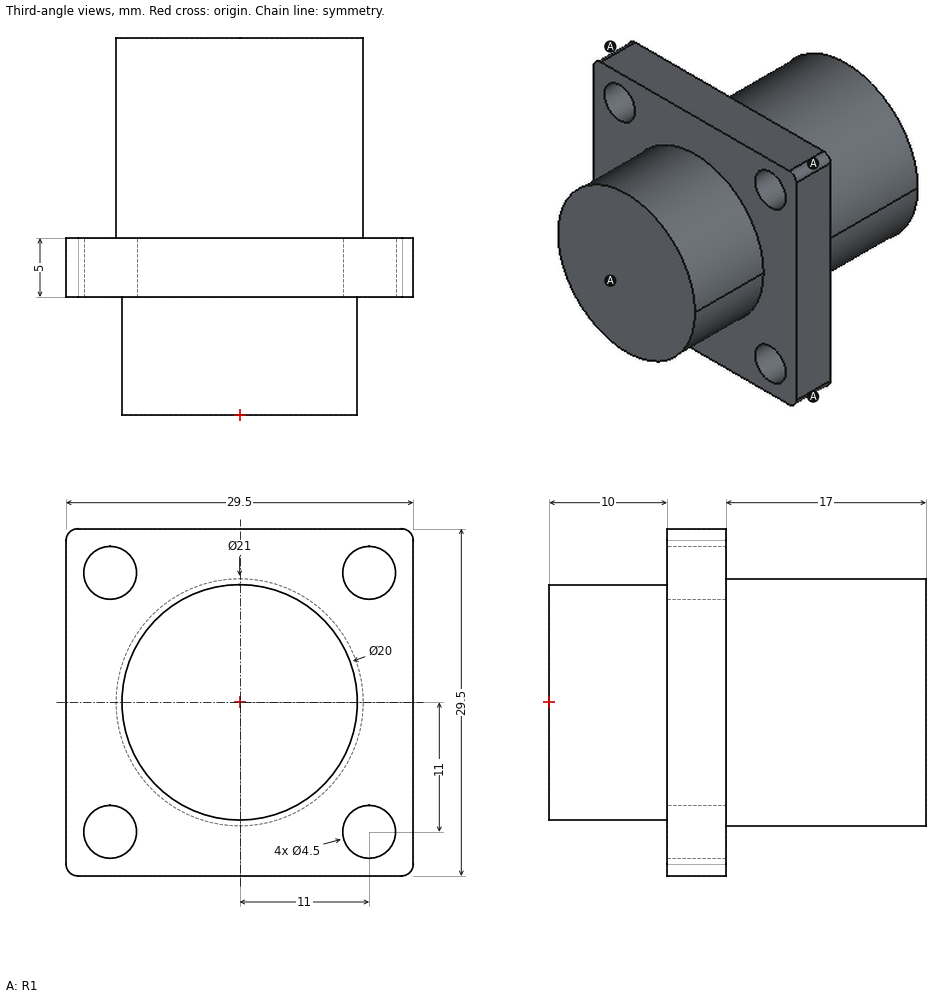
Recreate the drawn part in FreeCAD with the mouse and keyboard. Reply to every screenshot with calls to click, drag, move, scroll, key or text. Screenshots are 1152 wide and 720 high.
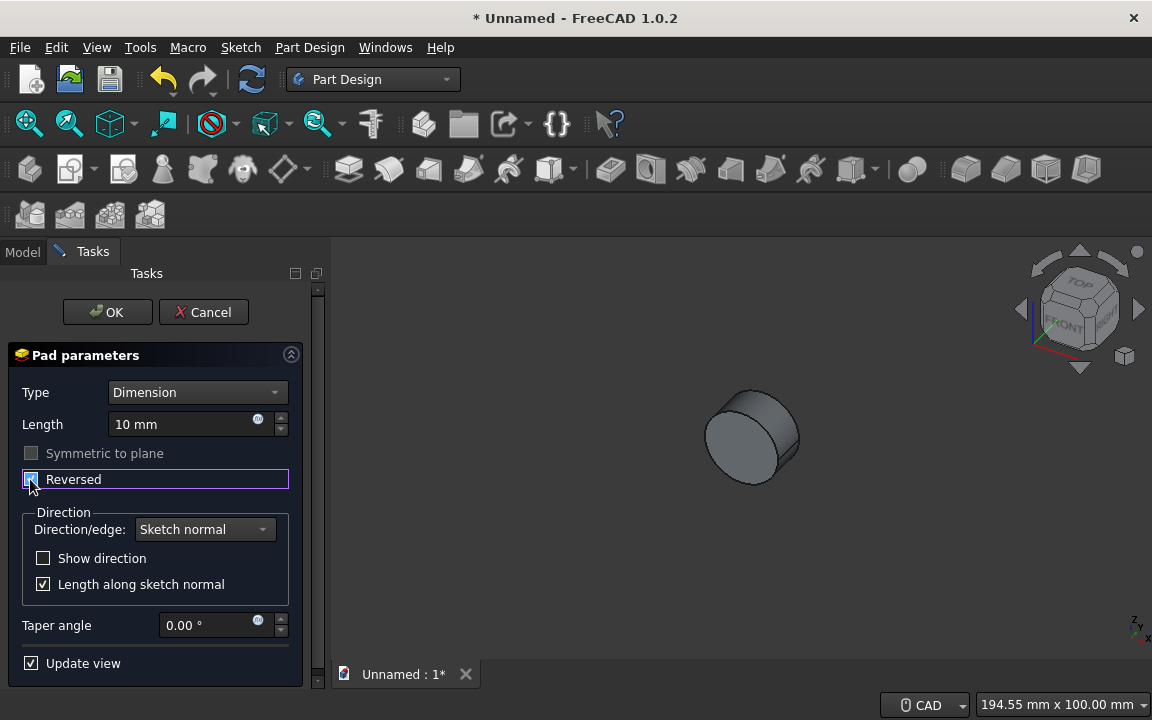
click(108, 312)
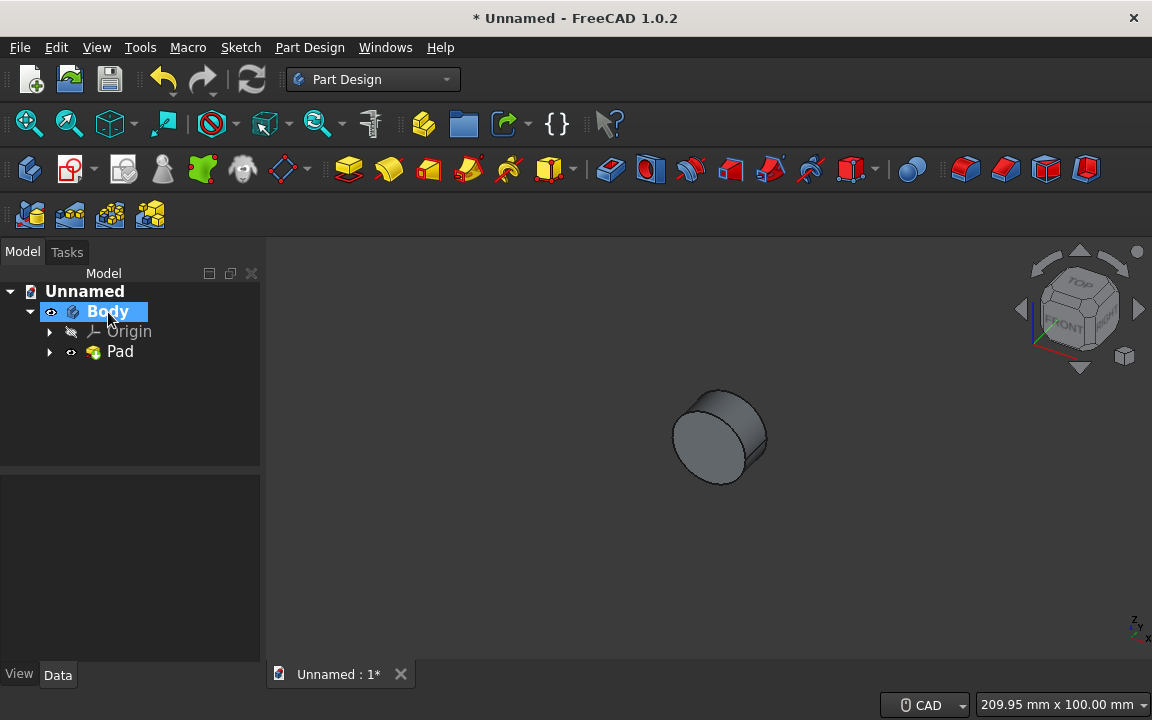
key(v)
key(f)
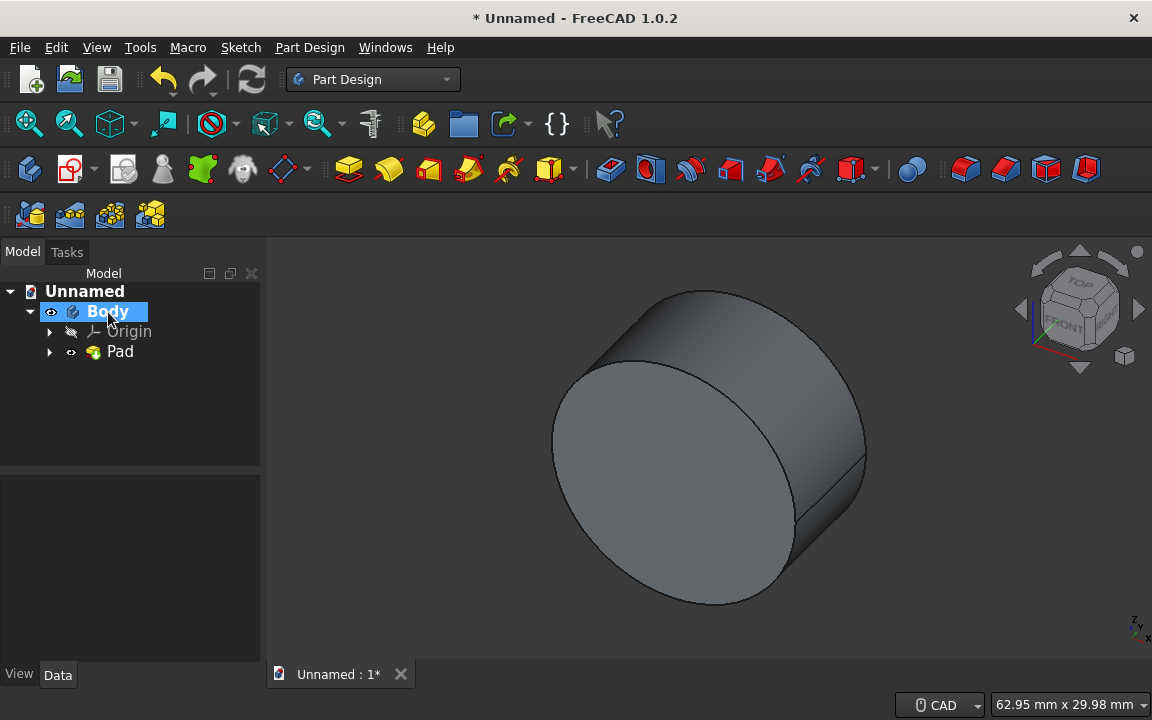
key(4)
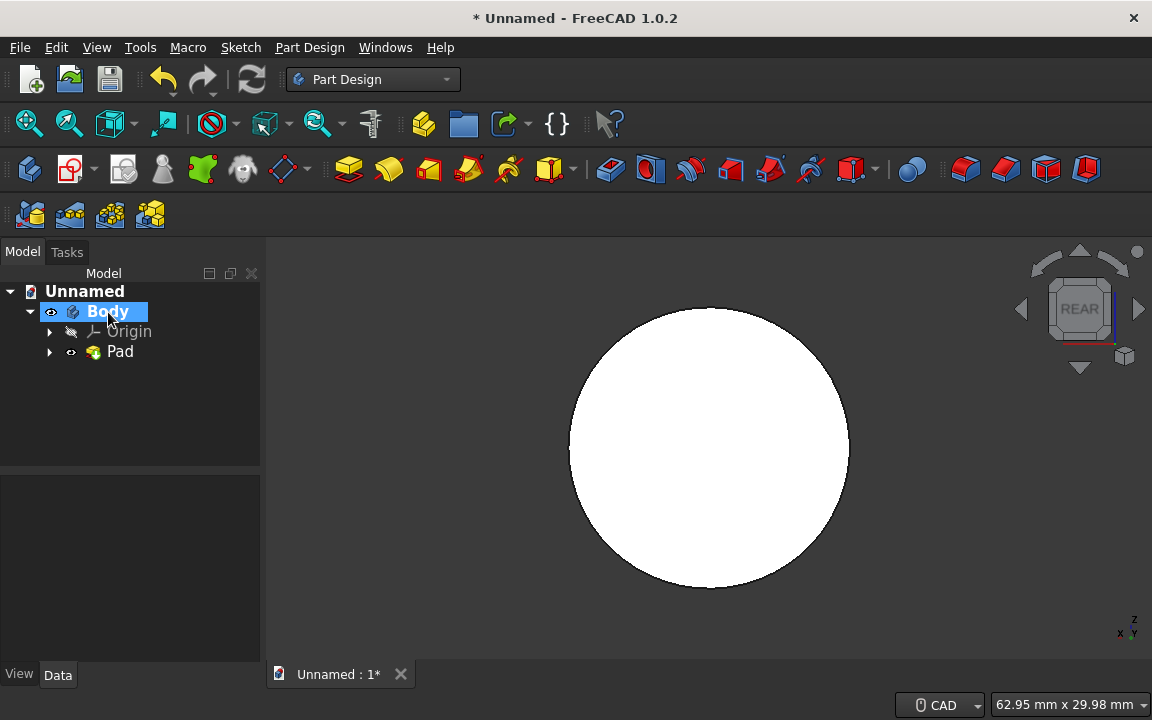
click(709, 447)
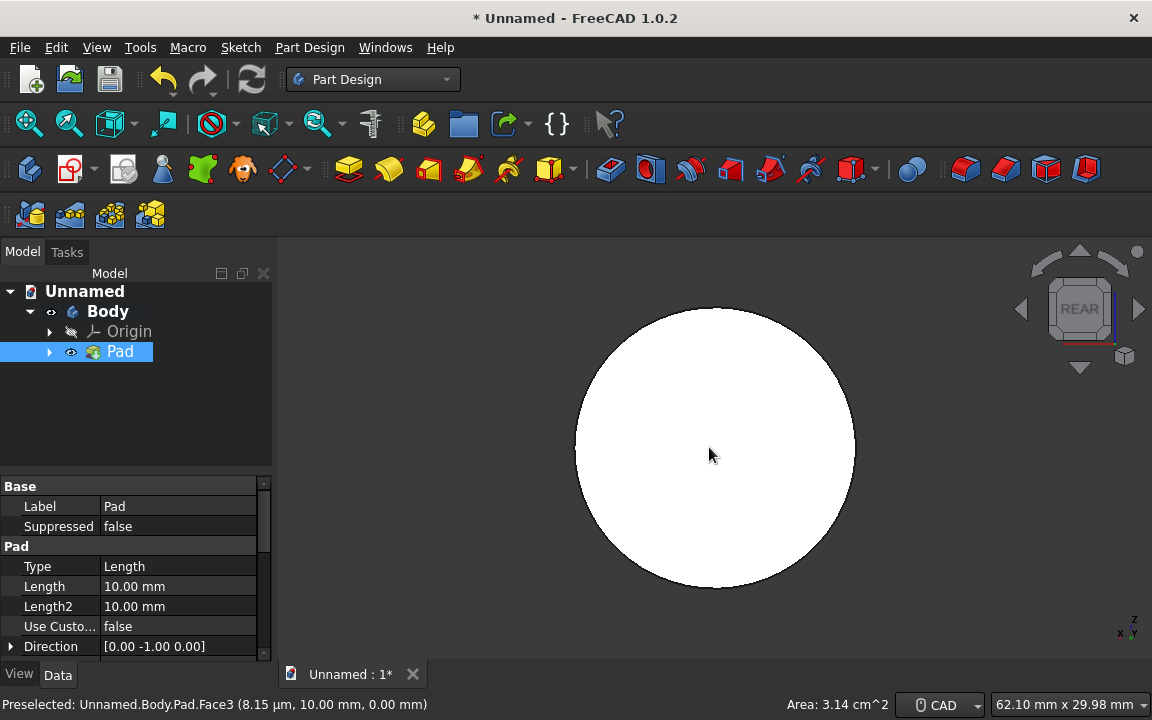
click(70, 170)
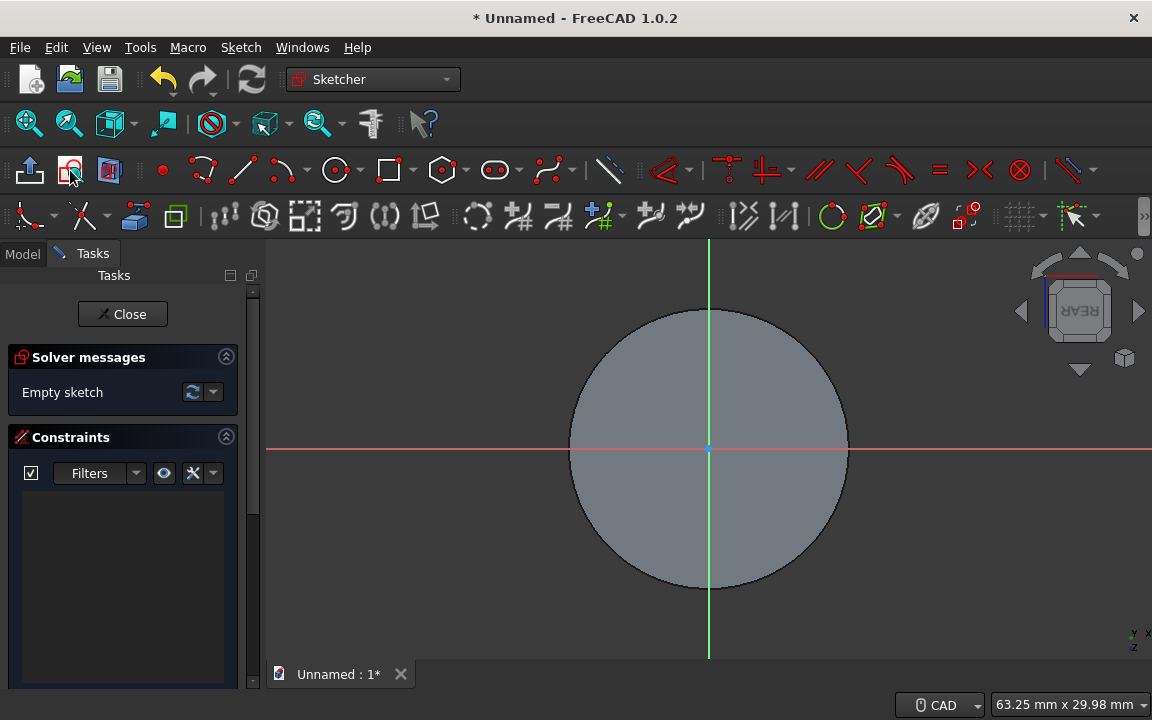
scroll(501, 449, down, 2)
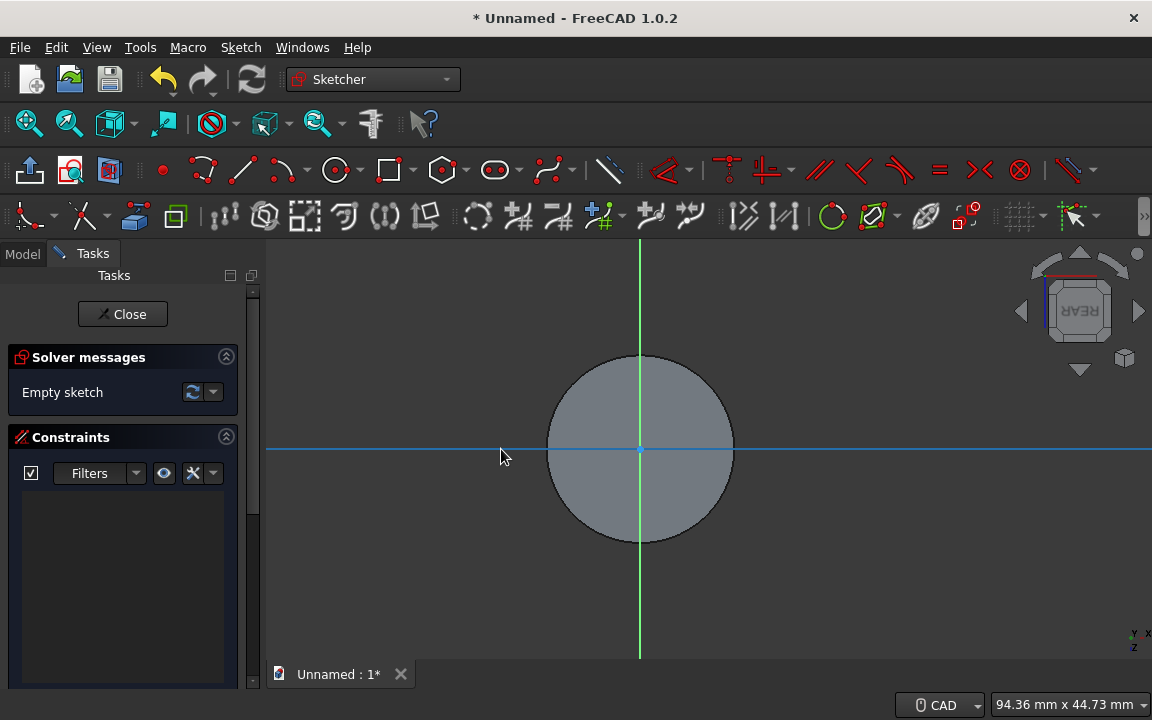
key(g)
key(v)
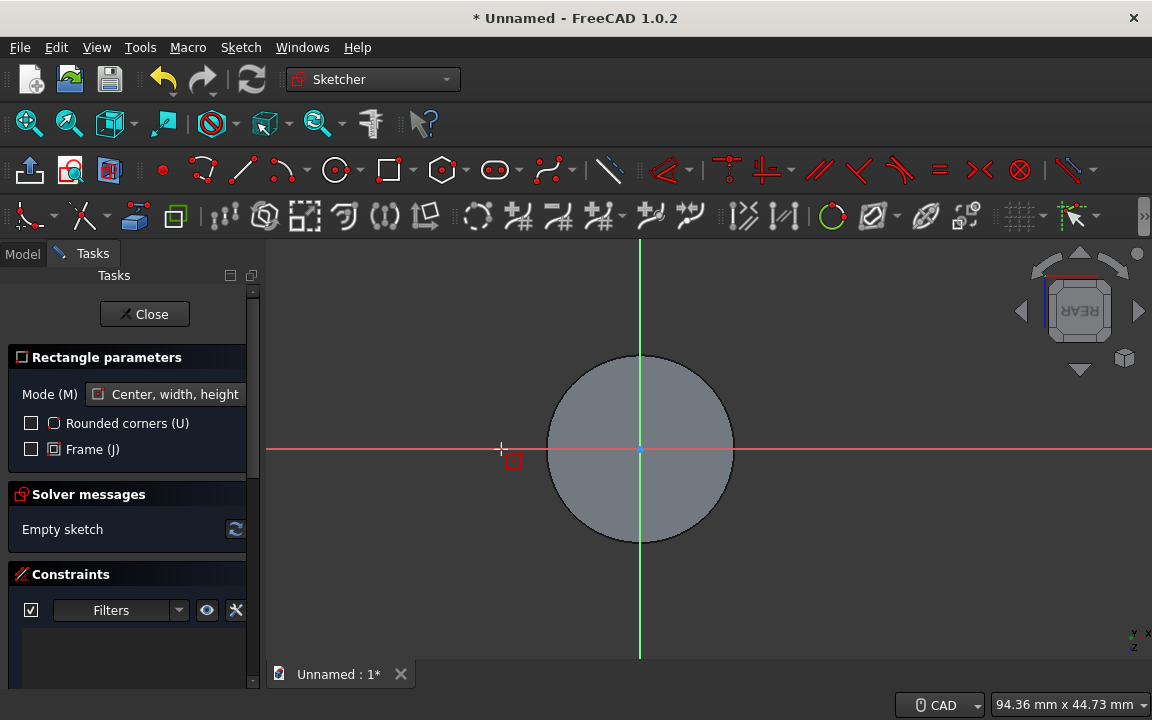
click(640, 449)
move(779, 311)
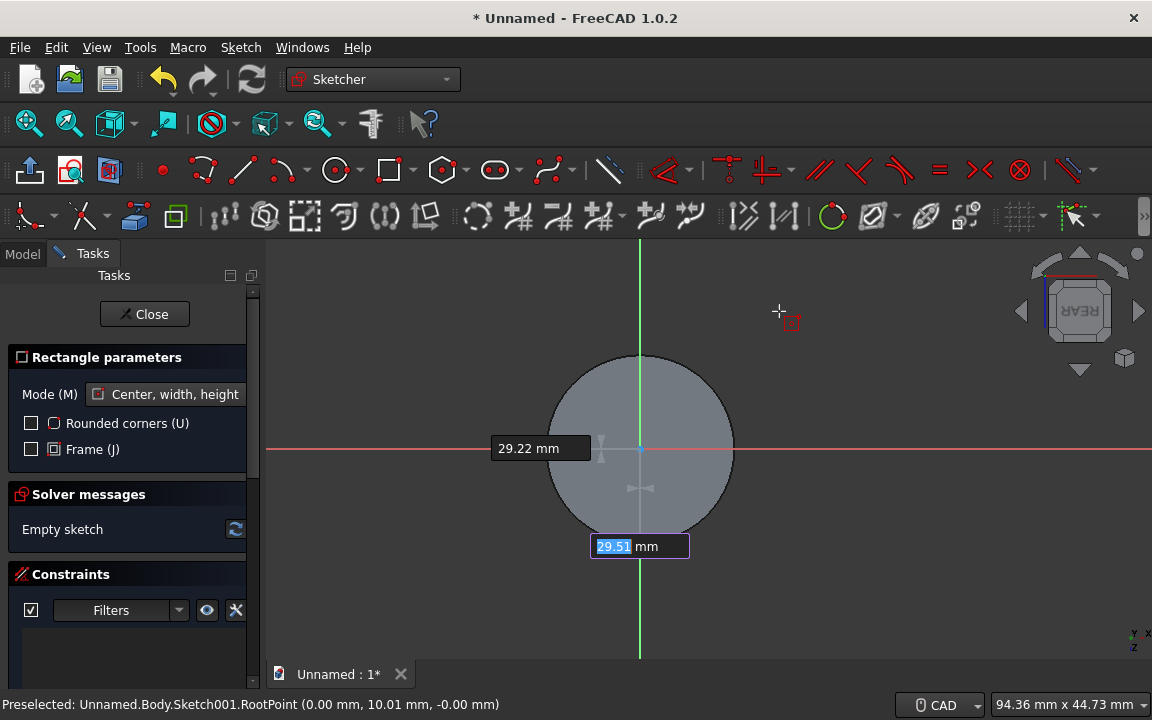
text(29.5)
key(Tab)
text(29.5)
key(Return)
key(Escape)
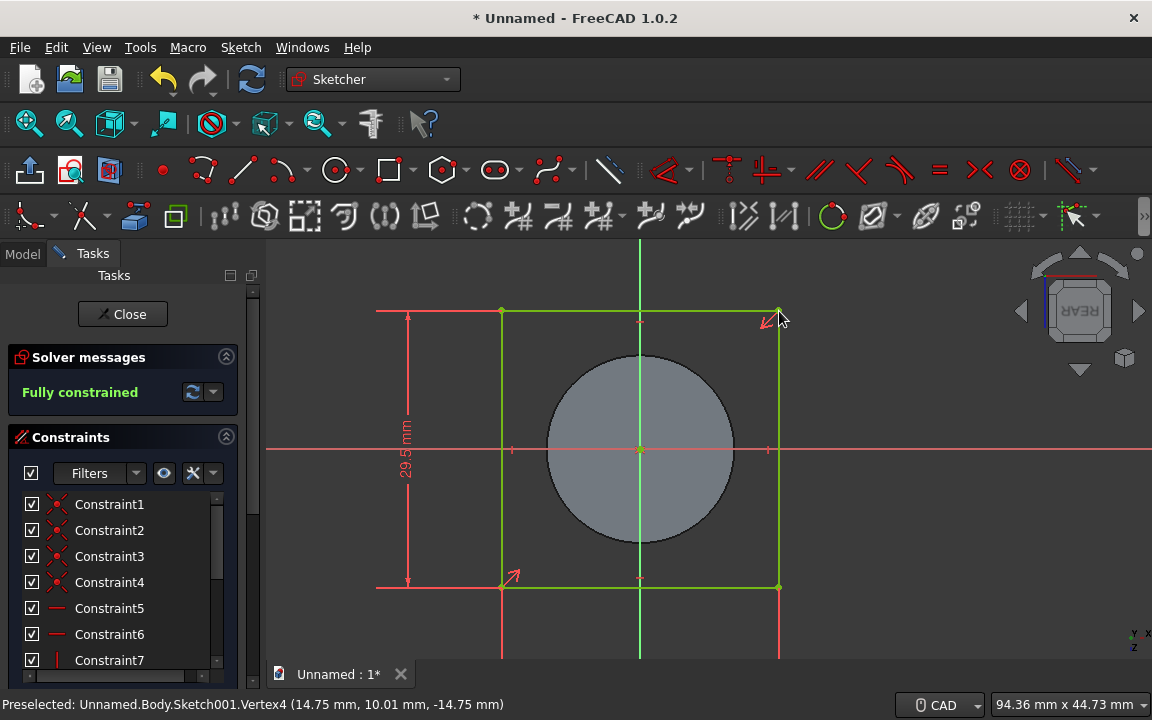
click(123, 314)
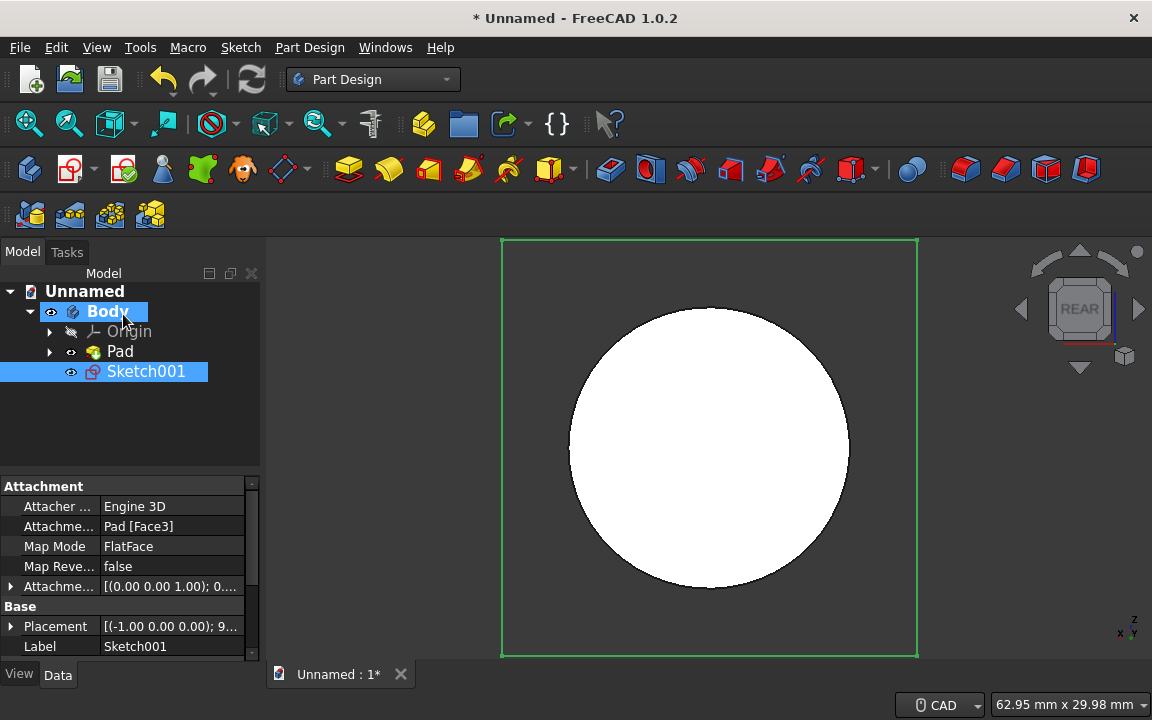
click(350, 170)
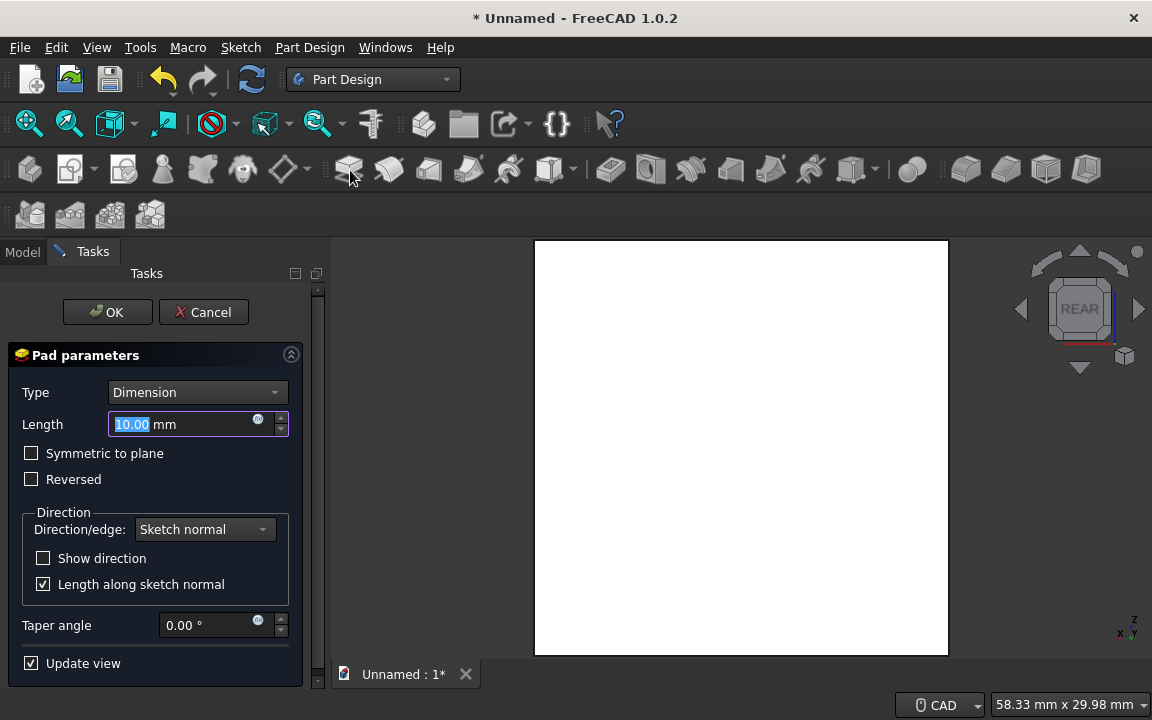
text(5)
key(Tab)